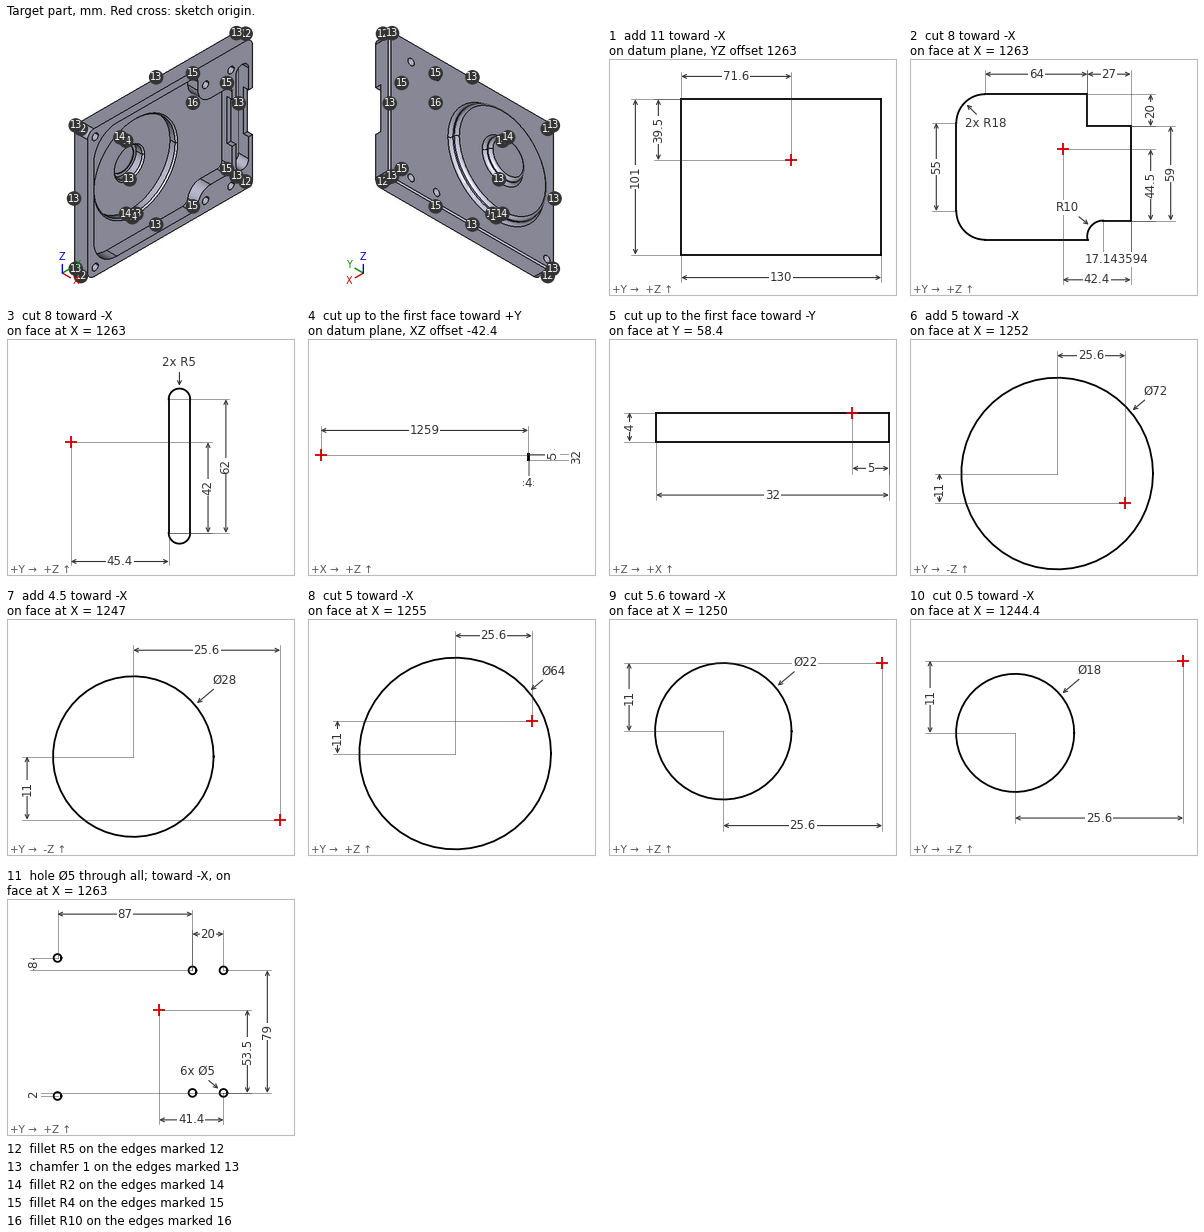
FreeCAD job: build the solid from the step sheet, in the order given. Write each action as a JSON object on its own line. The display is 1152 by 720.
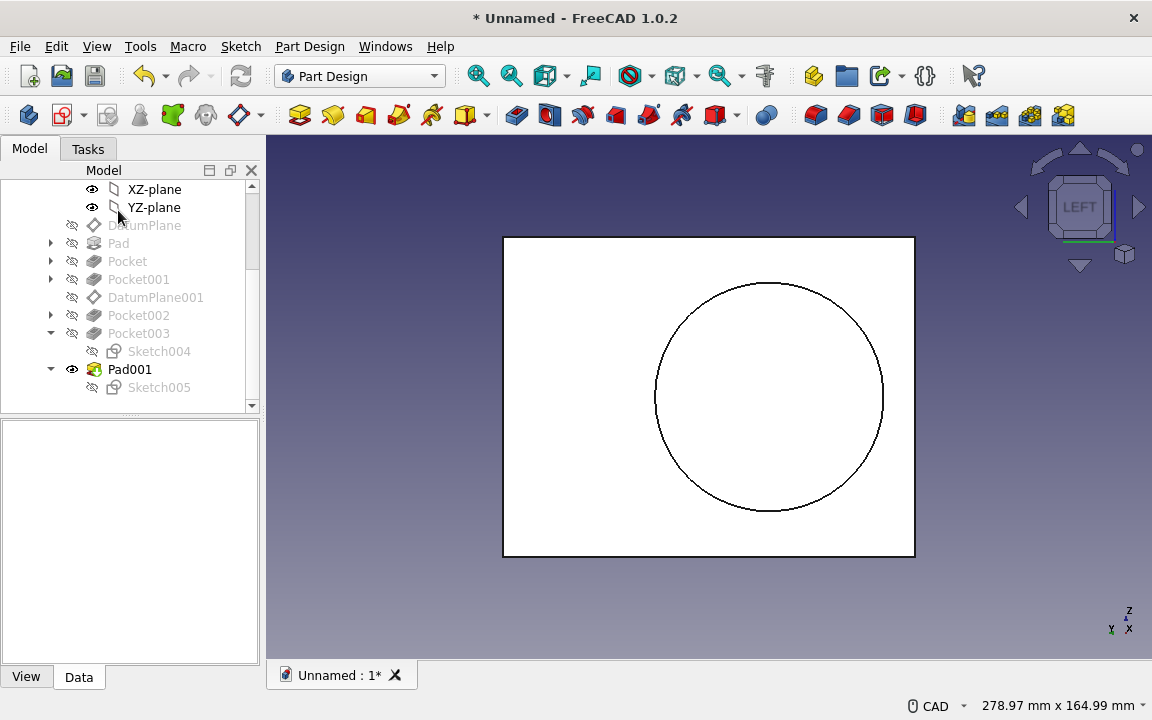
{"action": "left_click", "coordinate": [769, 396]}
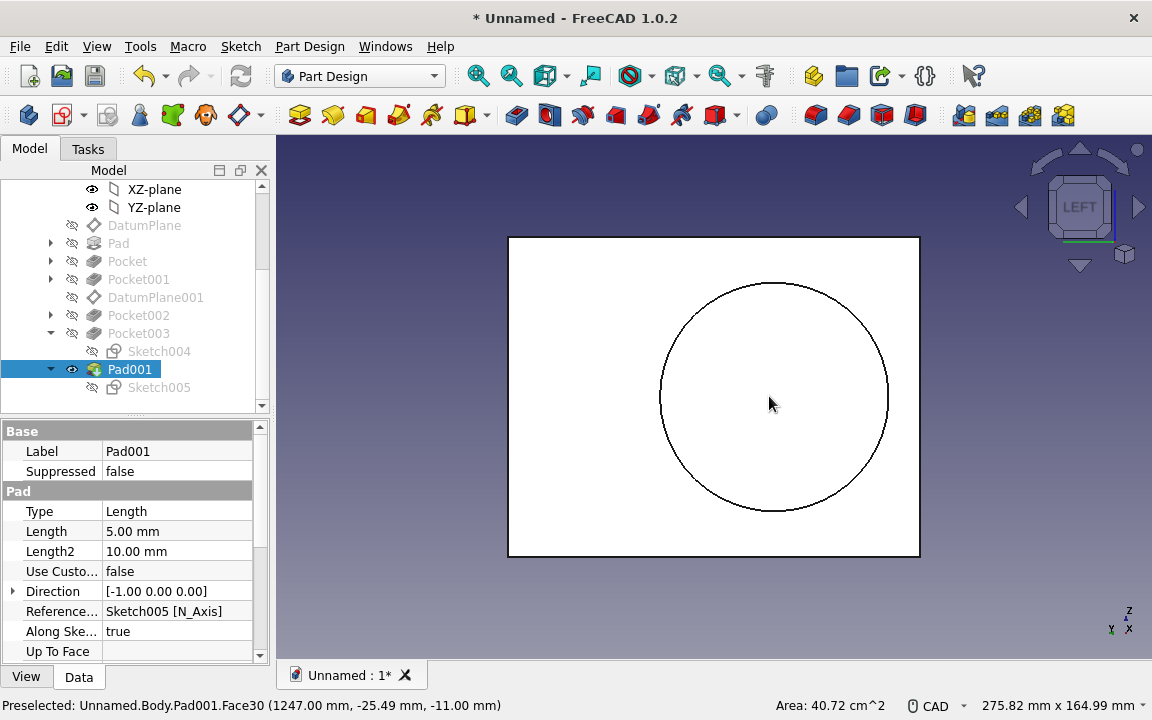
{"action": "left_click", "coordinate": [62, 116]}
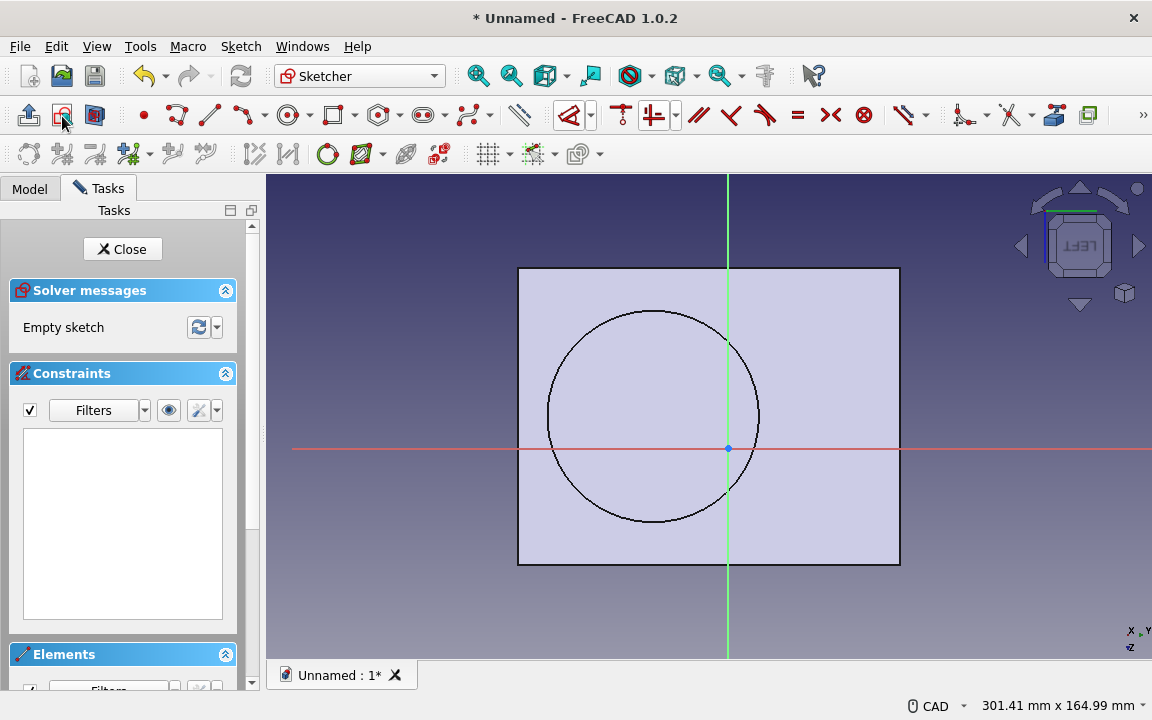
{"action": "scroll", "coordinate": [680, 416], "scroll_direction": "up", "scroll_amount": 7}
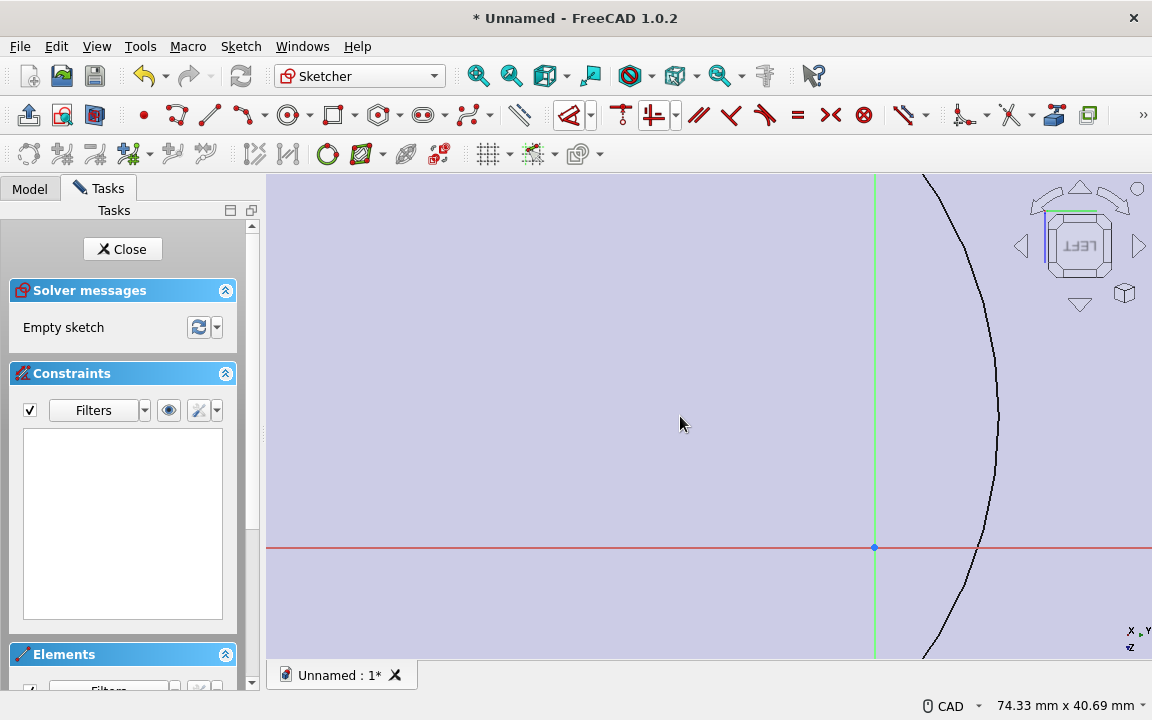
{"action": "left_click", "coordinate": [288, 116]}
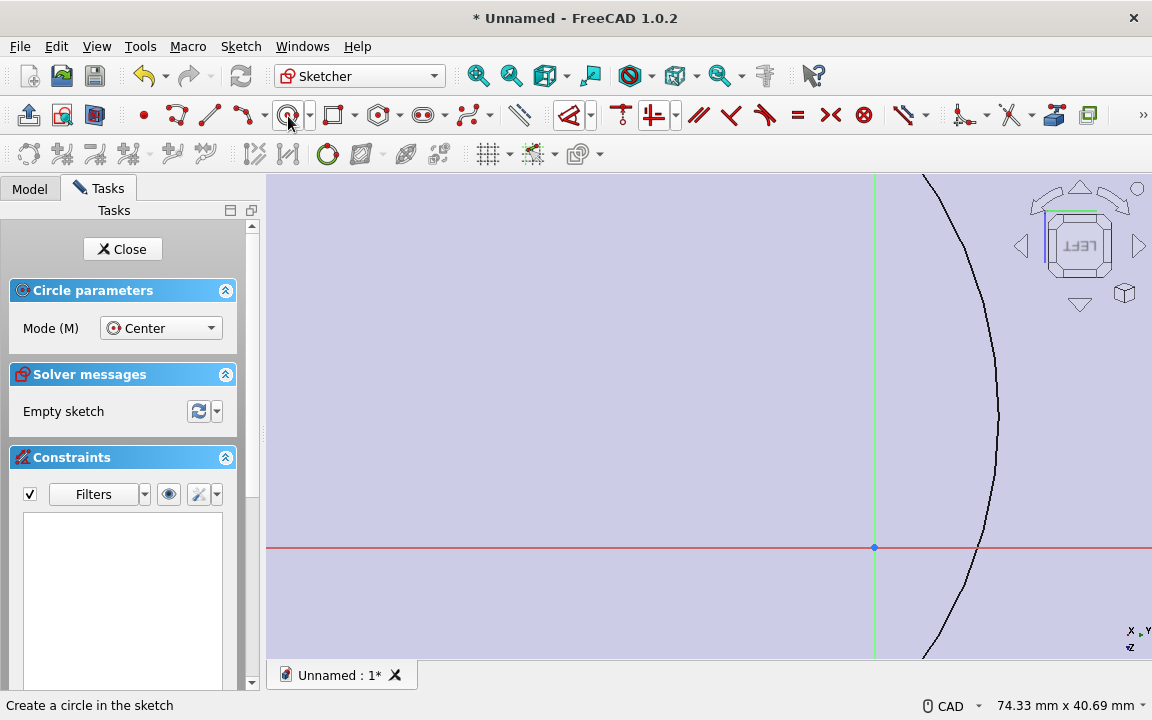
{"action": "left_click", "coordinate": [570, 416]}
{"action": "left_click", "coordinate": [688, 298]}
{"action": "key", "text": "Escape"}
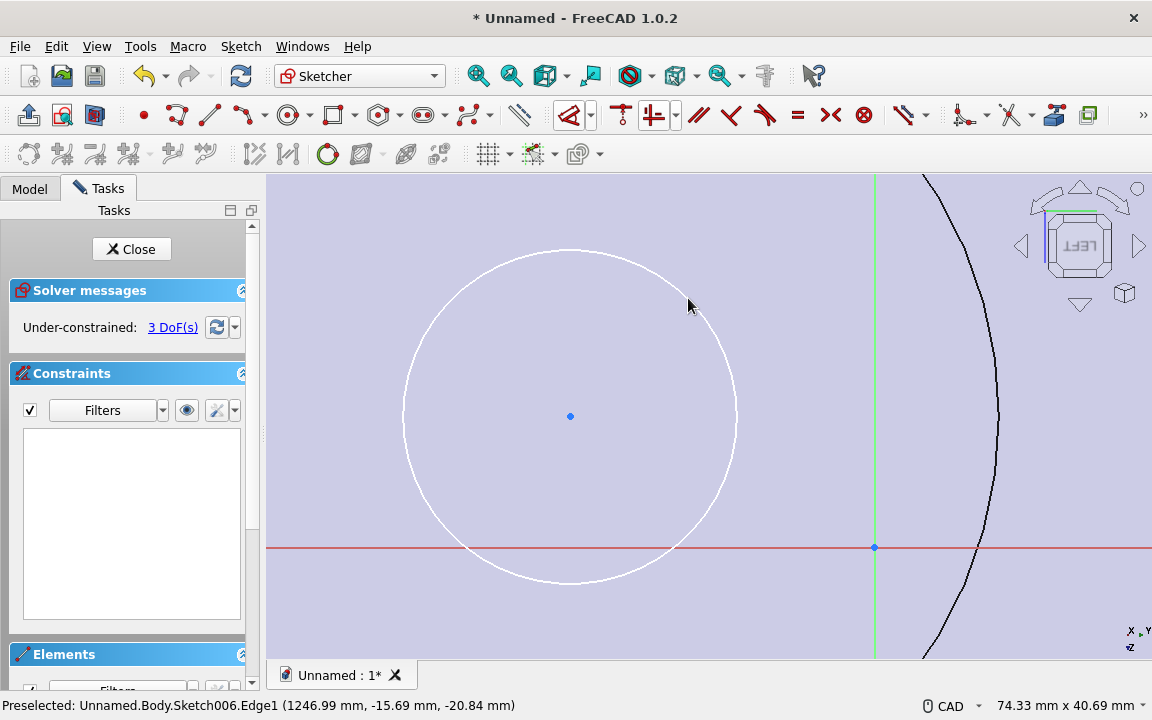
{"action": "left_click", "coordinate": [688, 299]}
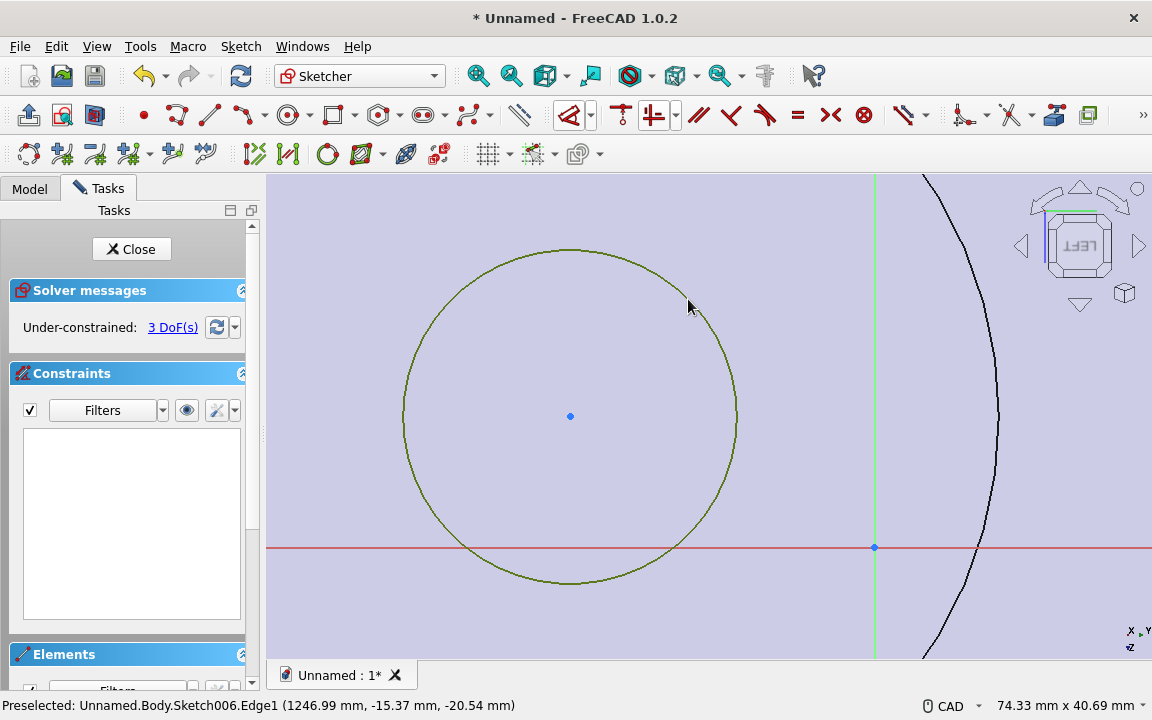
{"action": "left_click", "coordinate": [590, 116]}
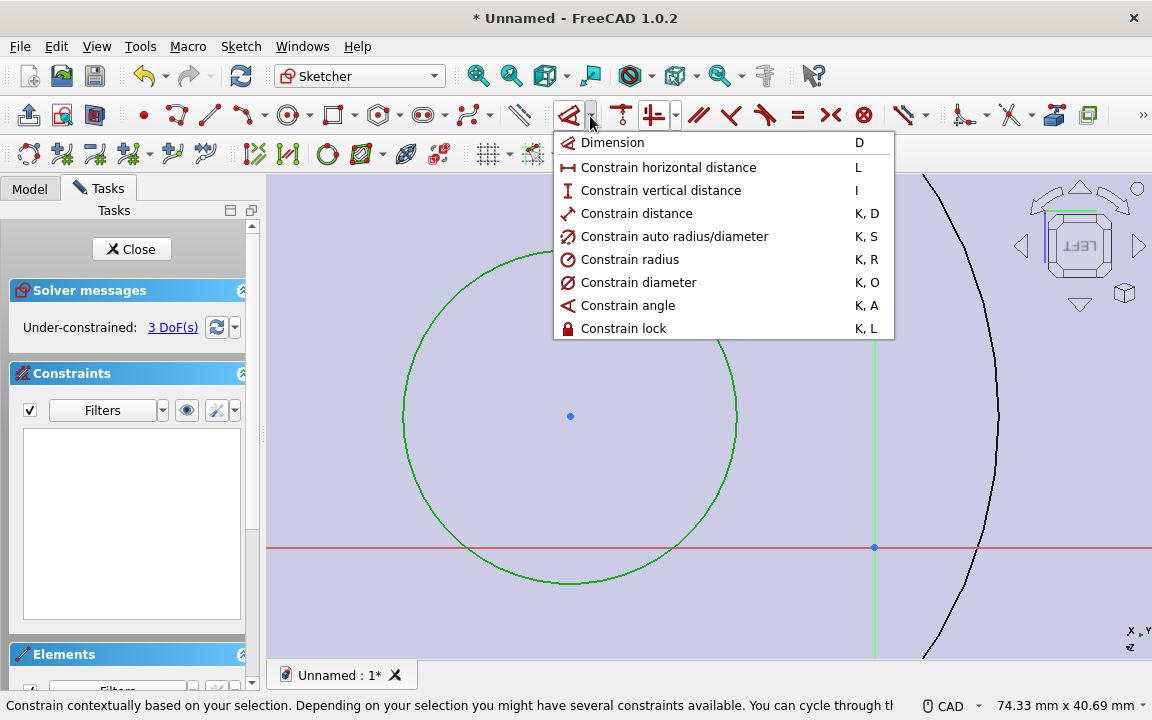
{"action": "left_click", "coordinate": [724, 282]}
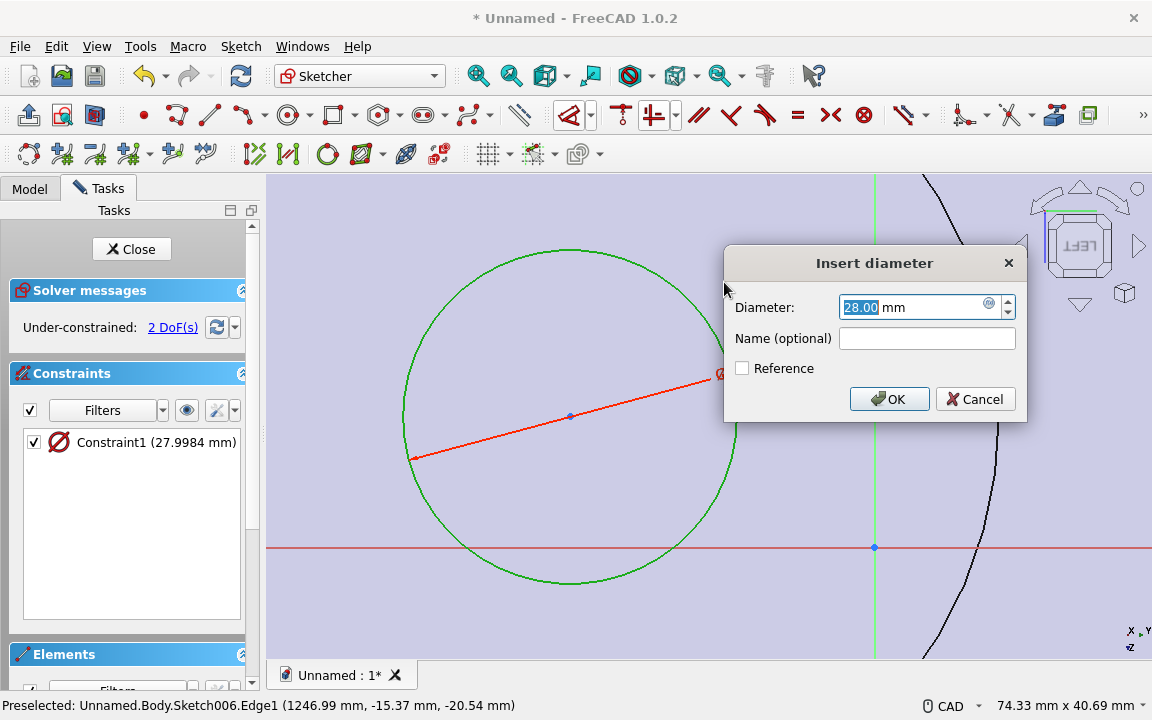
{"action": "type", "text": "28"}
{"action": "key", "text": "Return"}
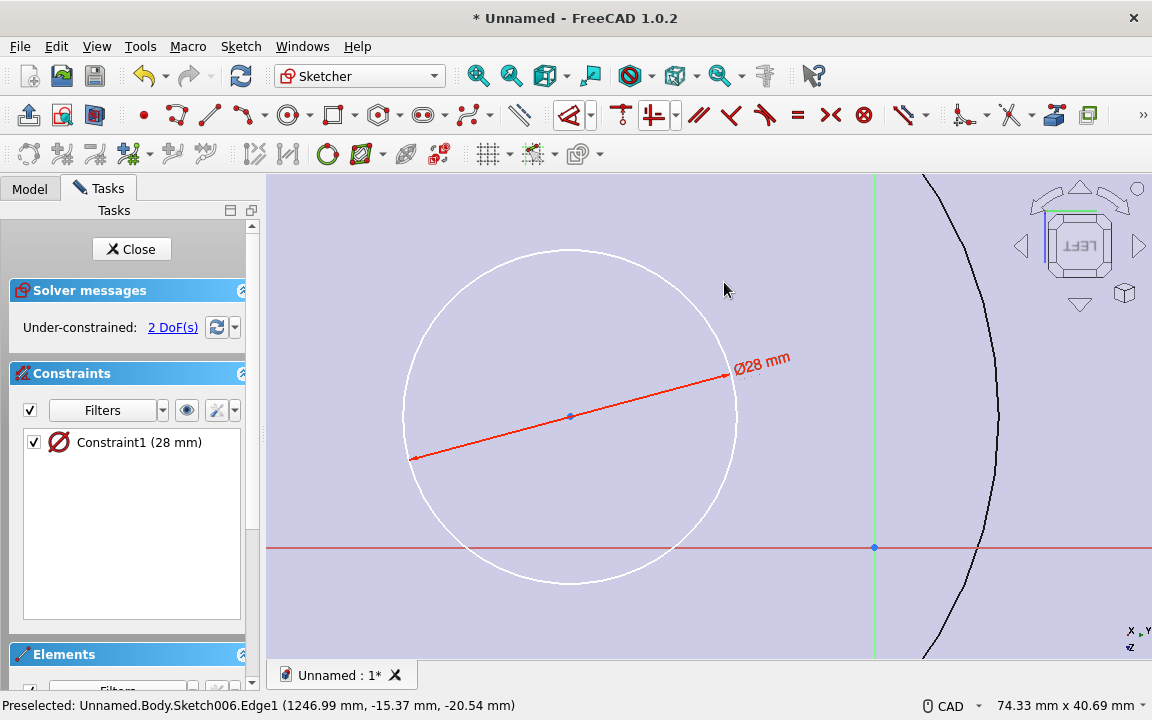
{"action": "left_click", "coordinate": [570, 417]}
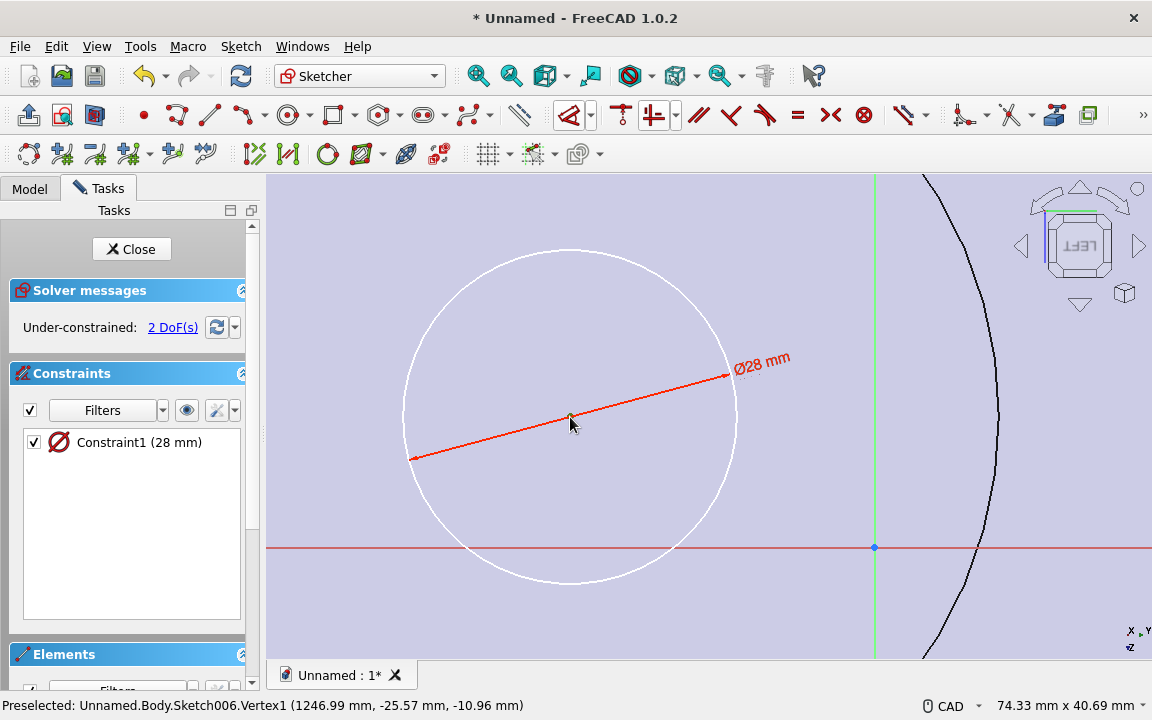
{"action": "key", "text": "i"}